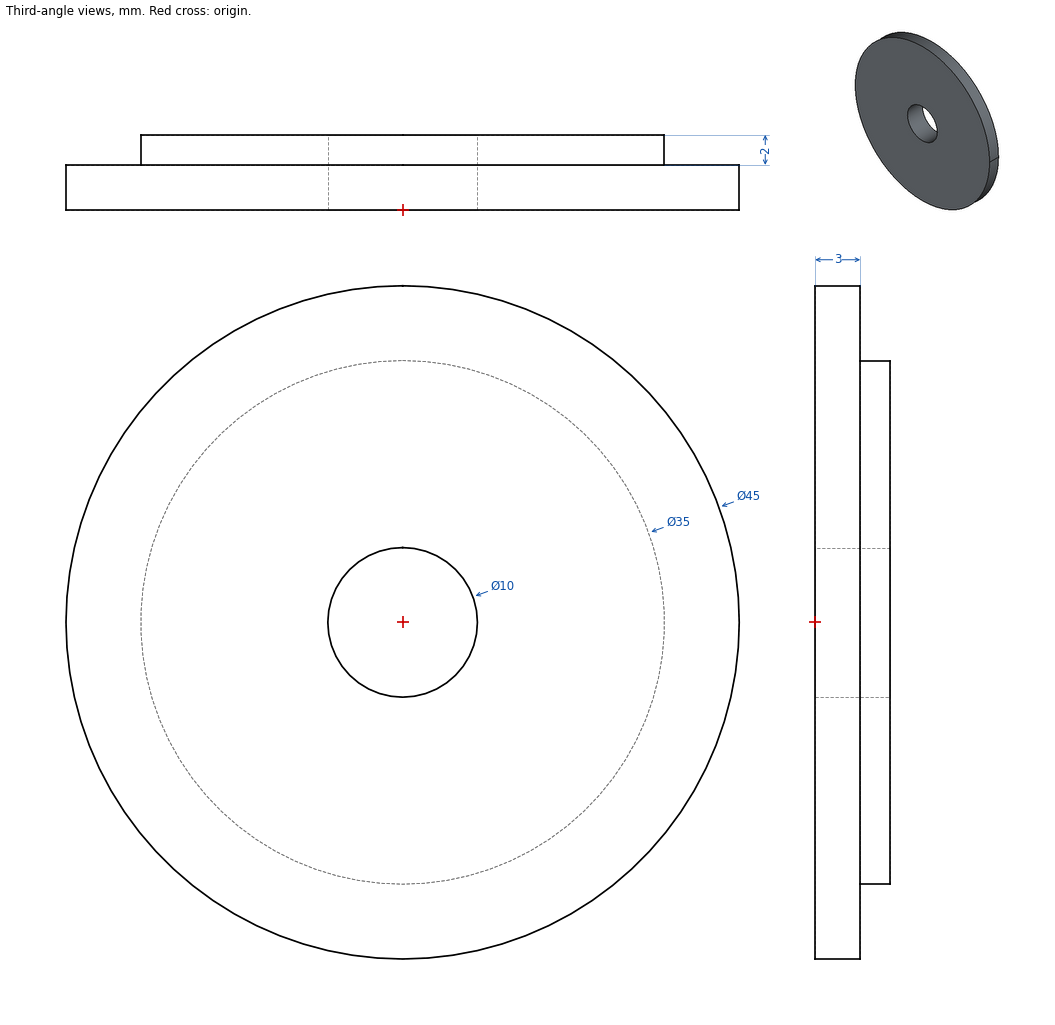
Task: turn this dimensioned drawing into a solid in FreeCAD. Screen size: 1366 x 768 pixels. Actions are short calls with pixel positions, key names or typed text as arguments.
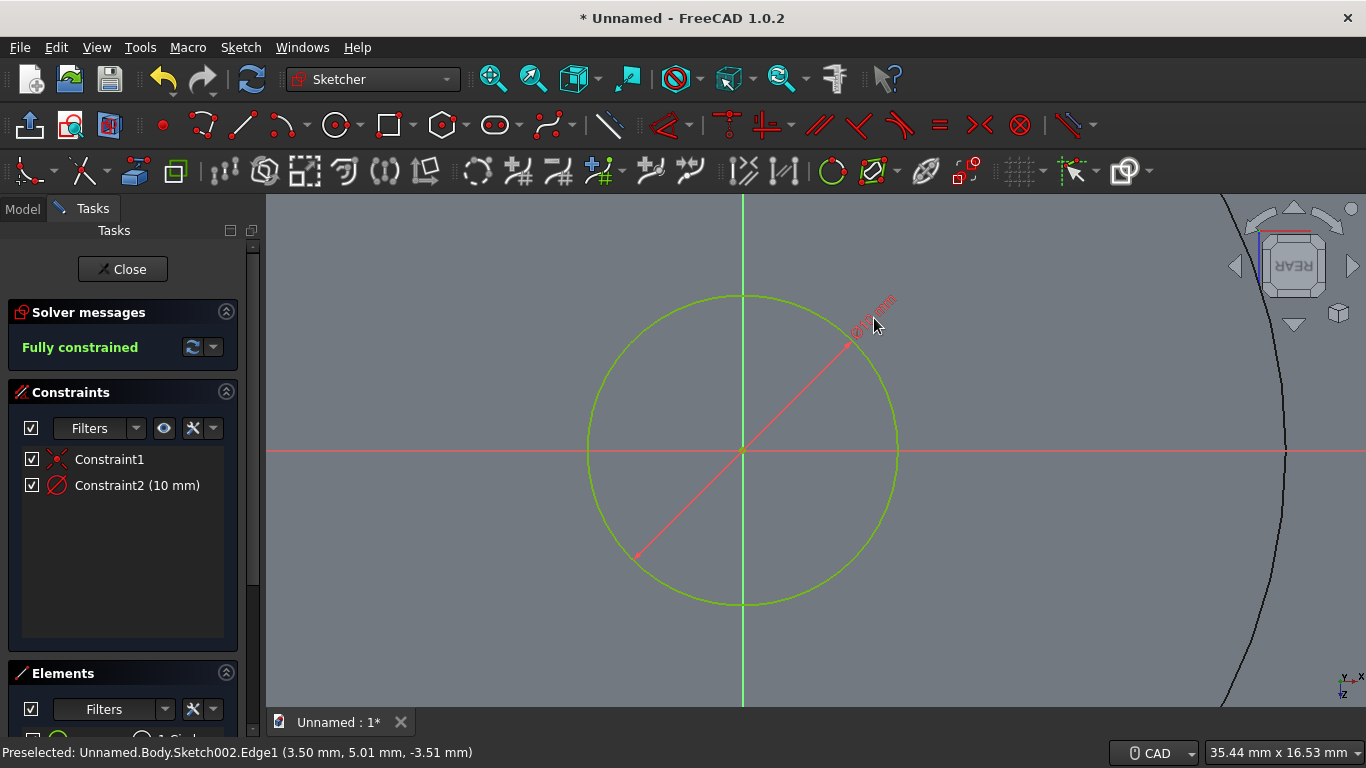
click(123, 269)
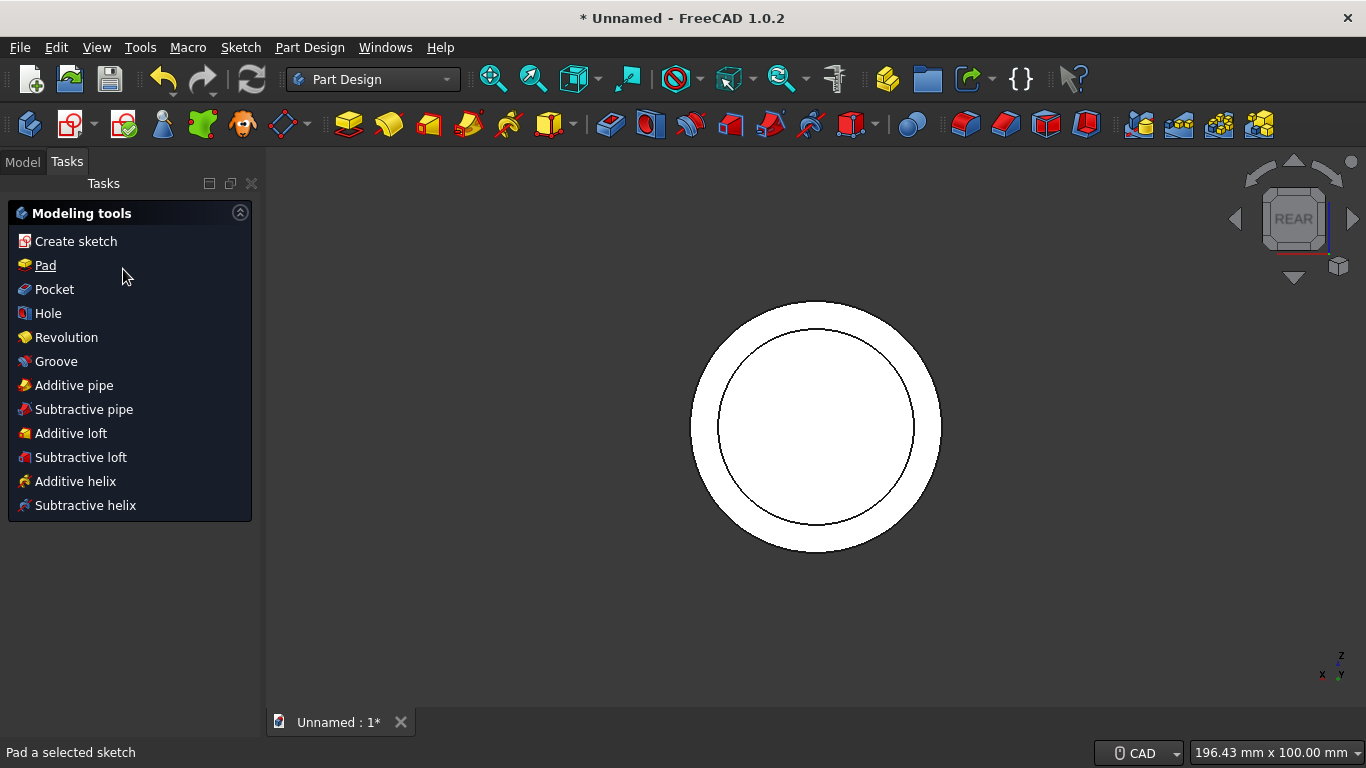
click(612, 124)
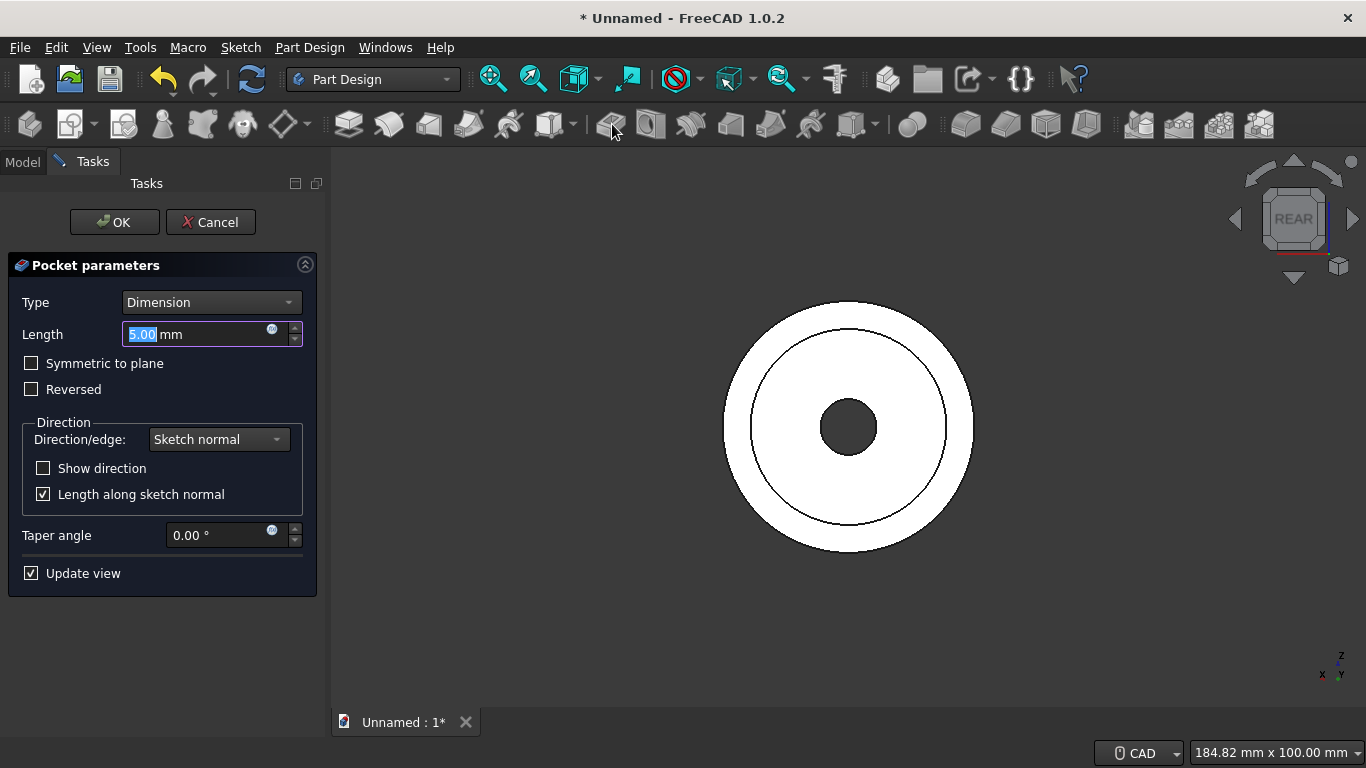
click(212, 302)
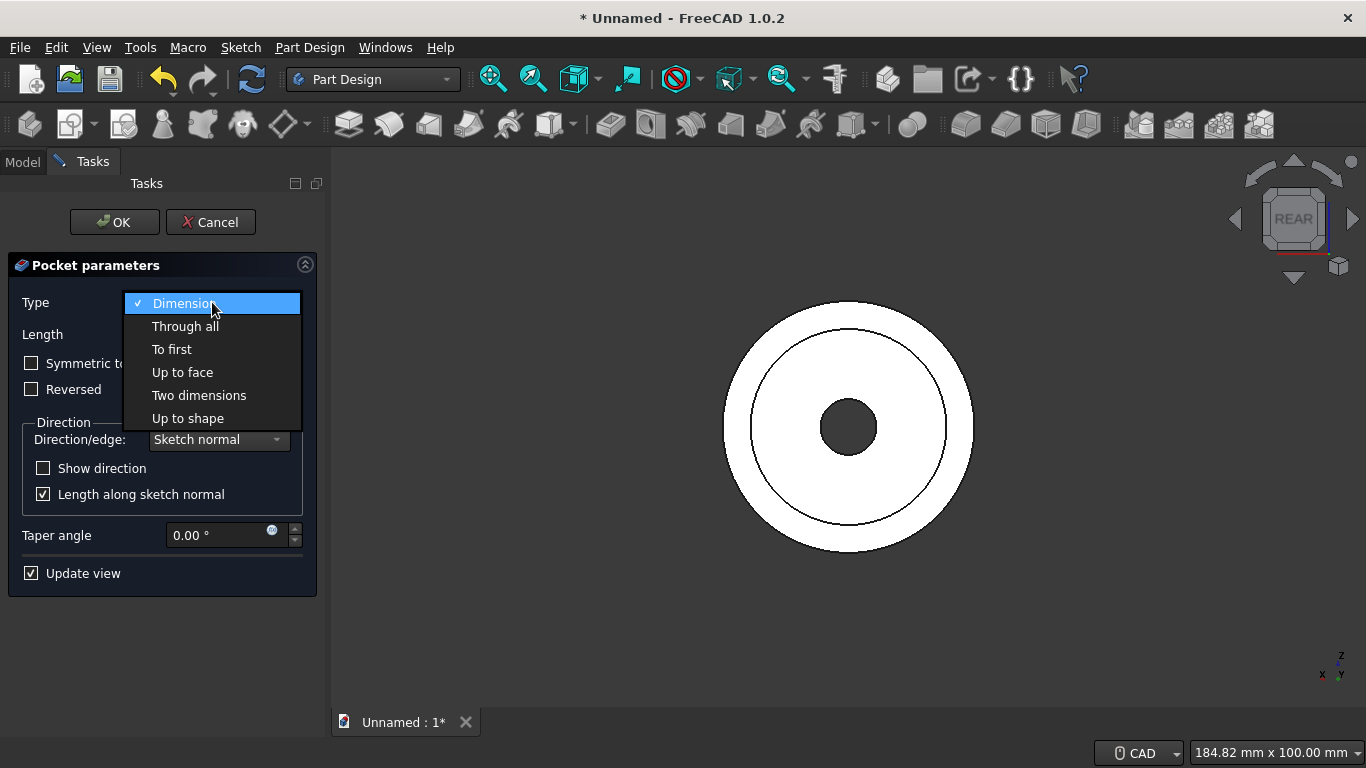
click(212, 326)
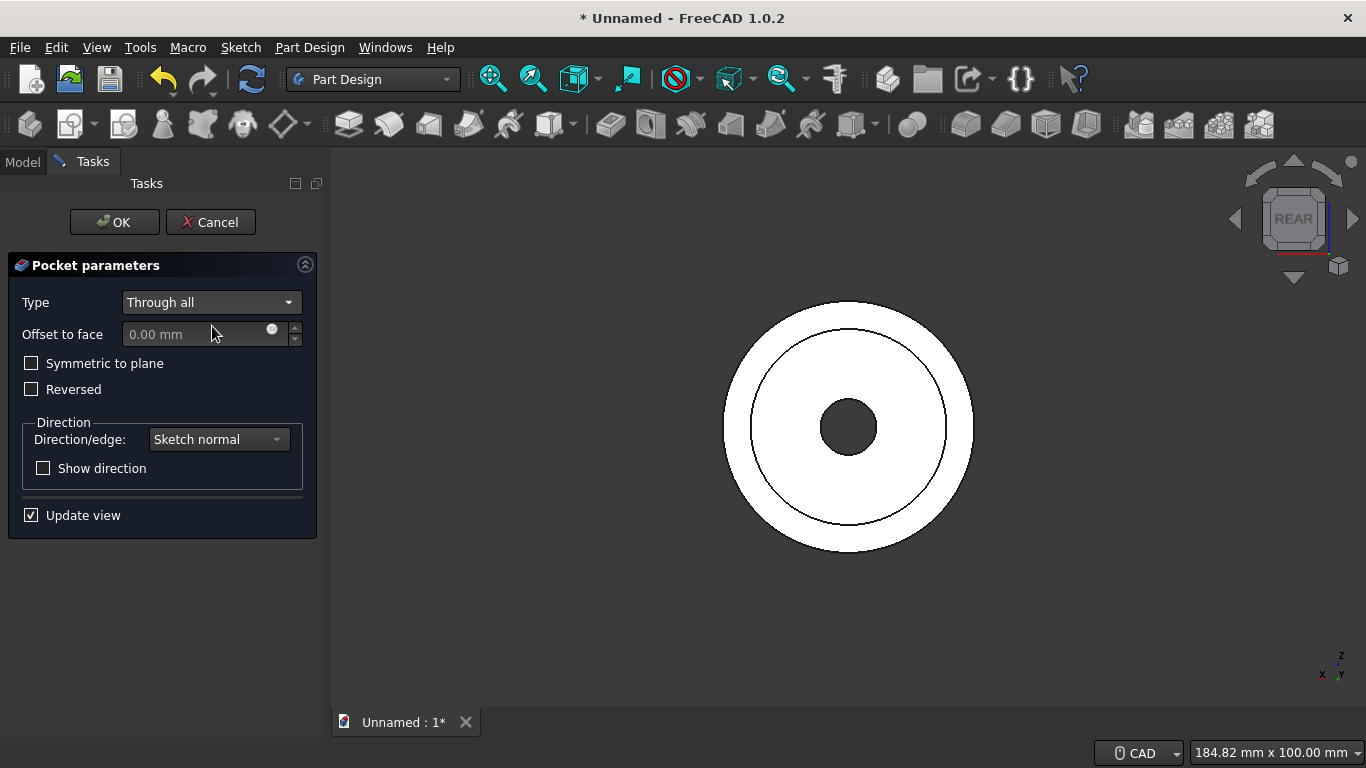
click(115, 222)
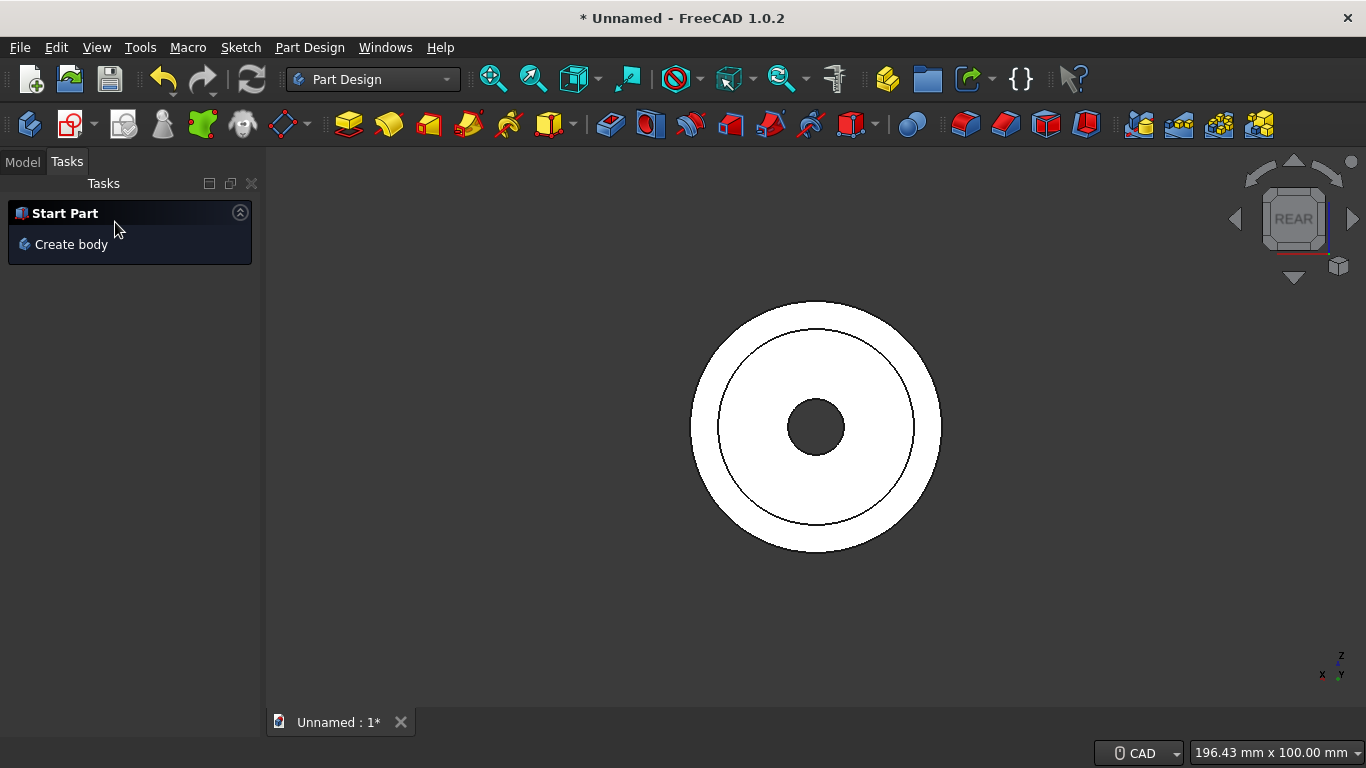
key(0)